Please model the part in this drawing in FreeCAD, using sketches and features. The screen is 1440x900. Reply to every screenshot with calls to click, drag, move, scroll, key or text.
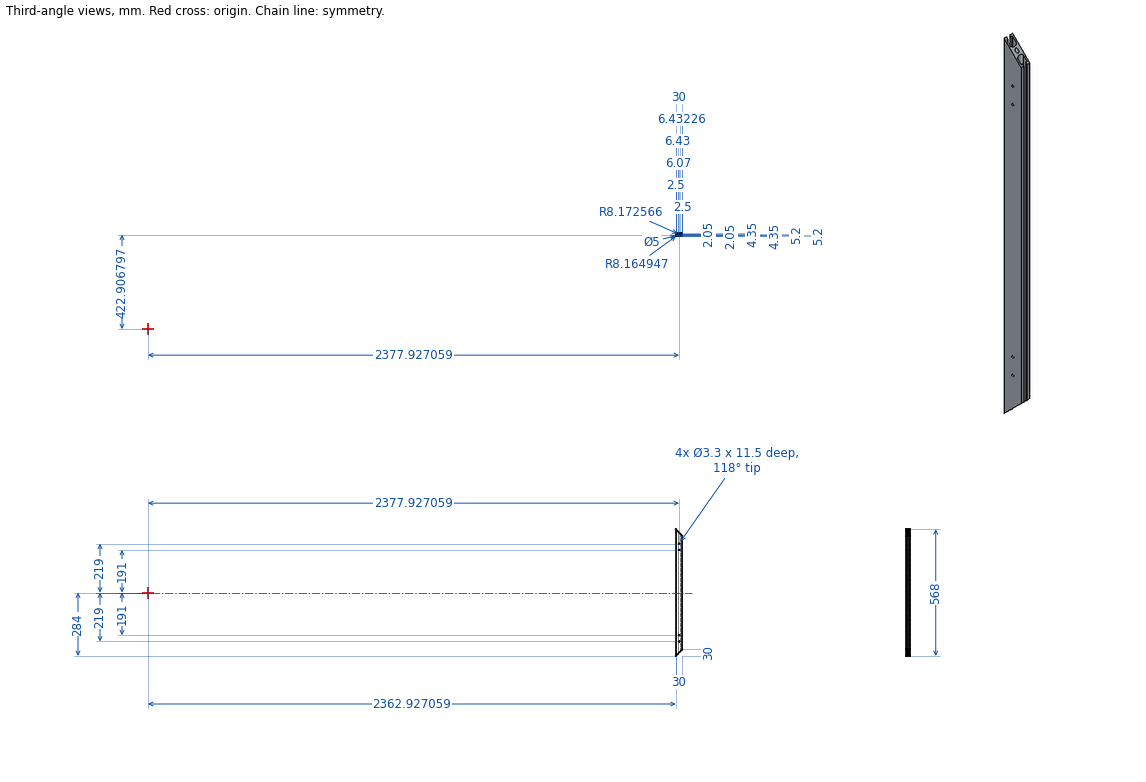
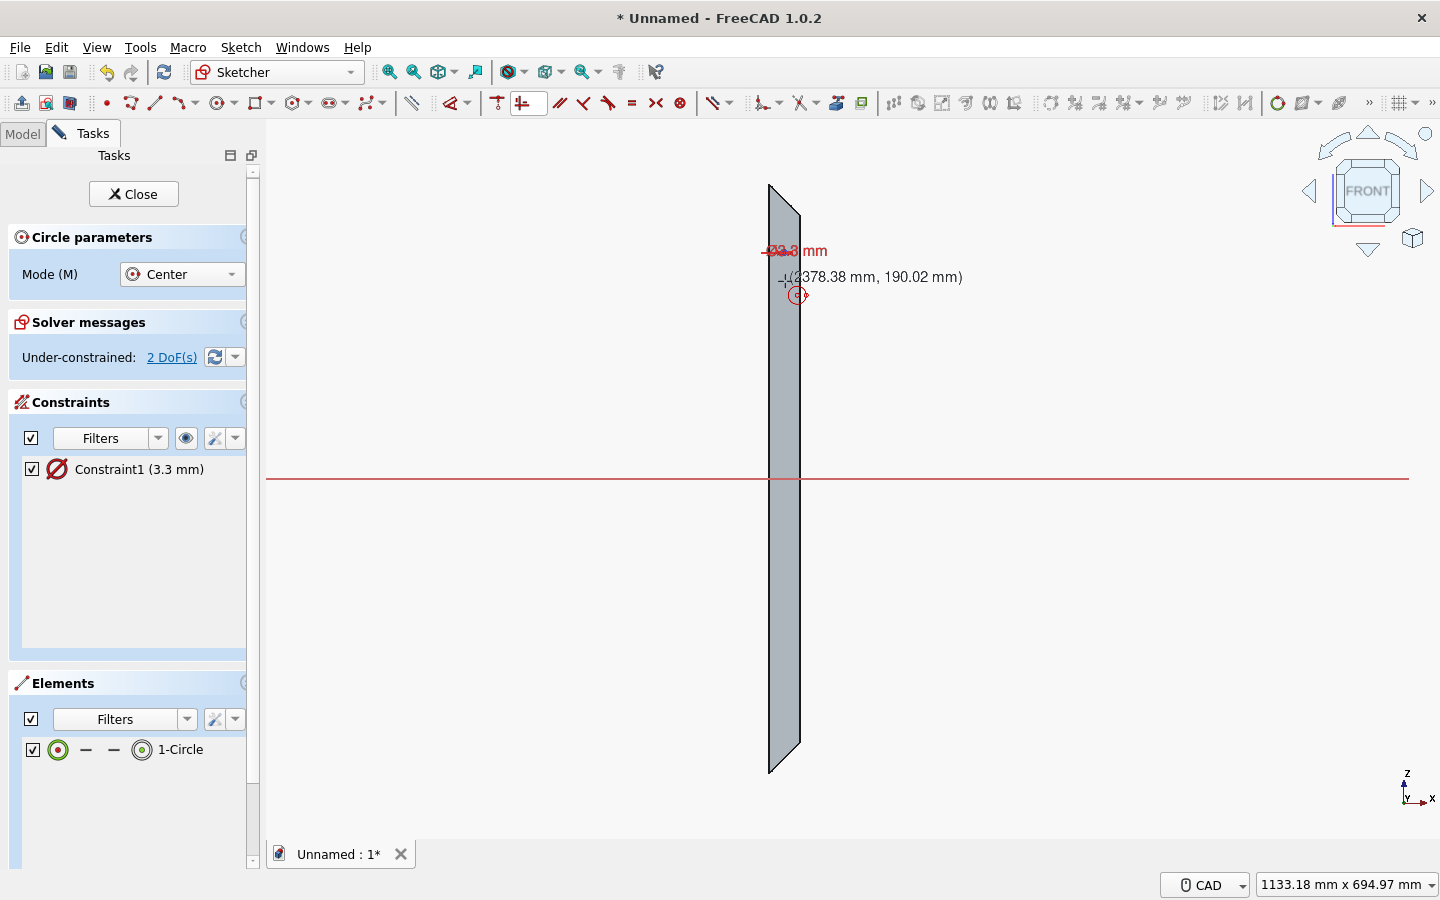
click(785, 281)
move(786, 280)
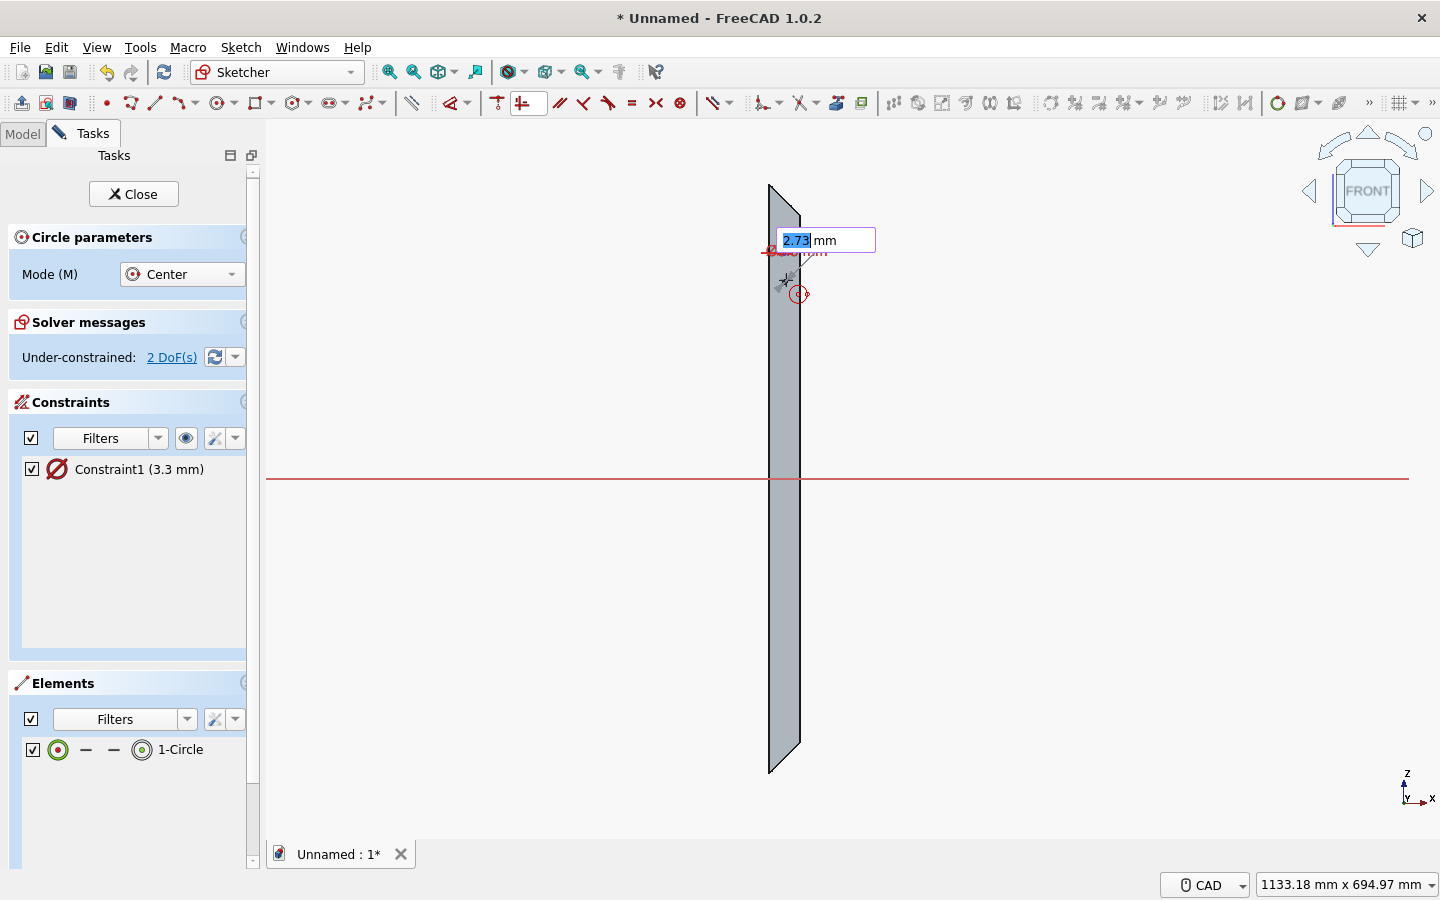
text(3.3)
key(Return)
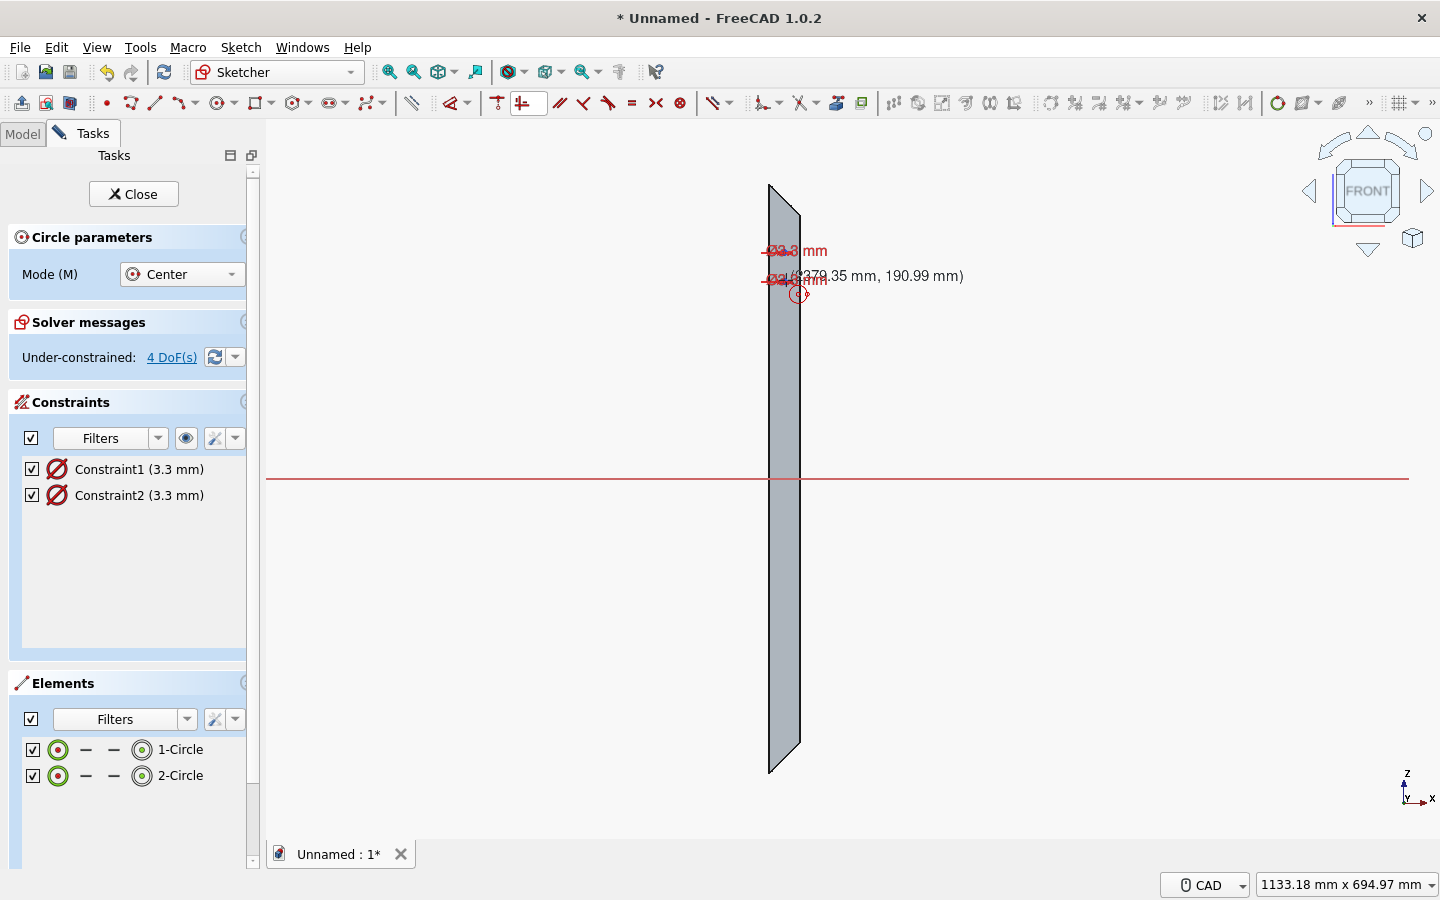
scroll(785, 677, up, 13)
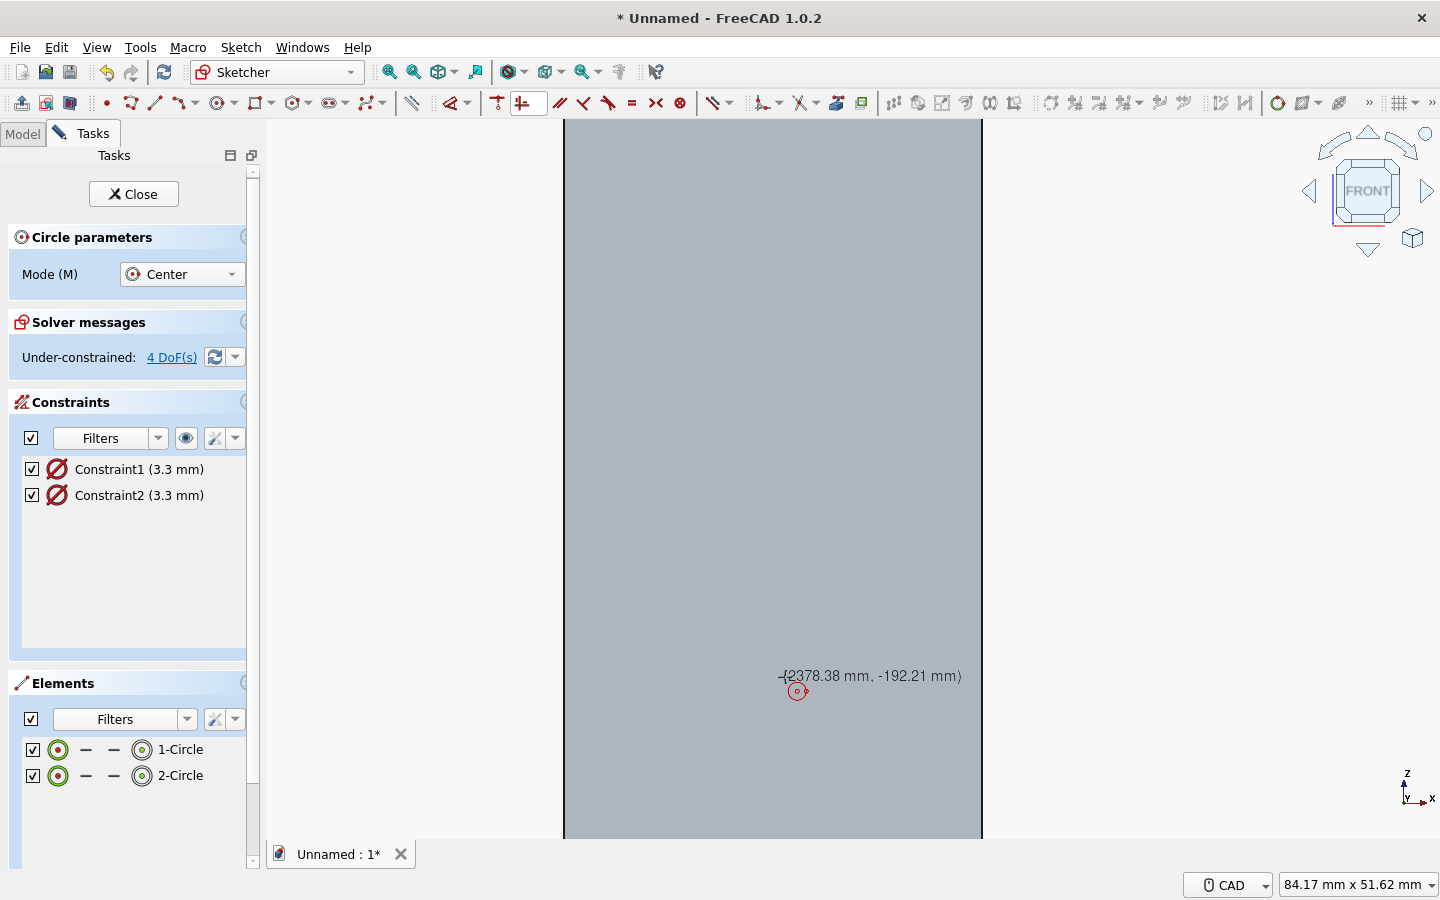
scroll(785, 678, down, 13)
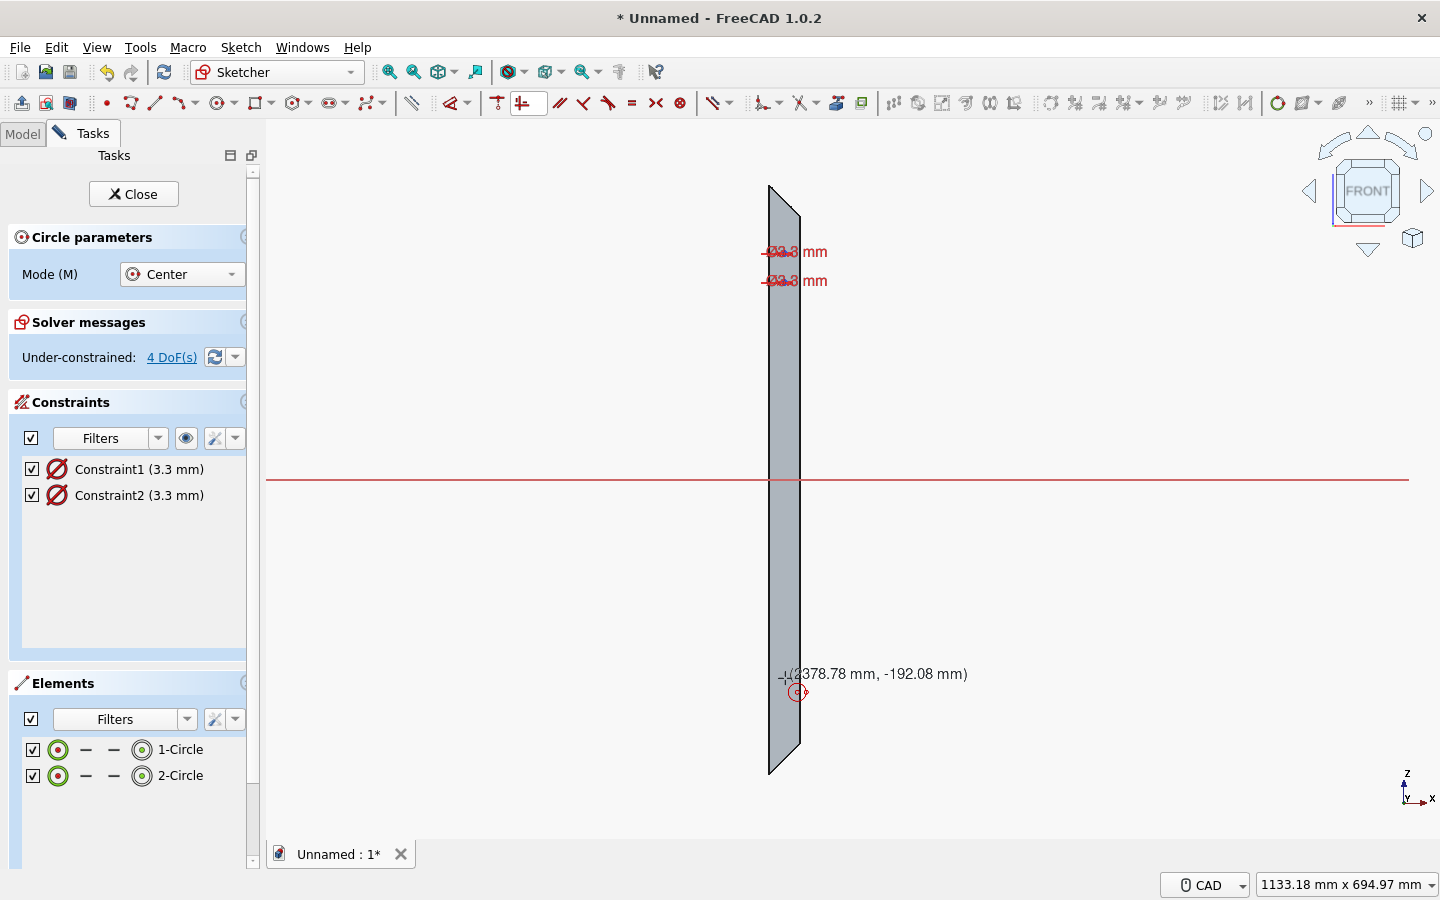
click(785, 678)
move(786, 676)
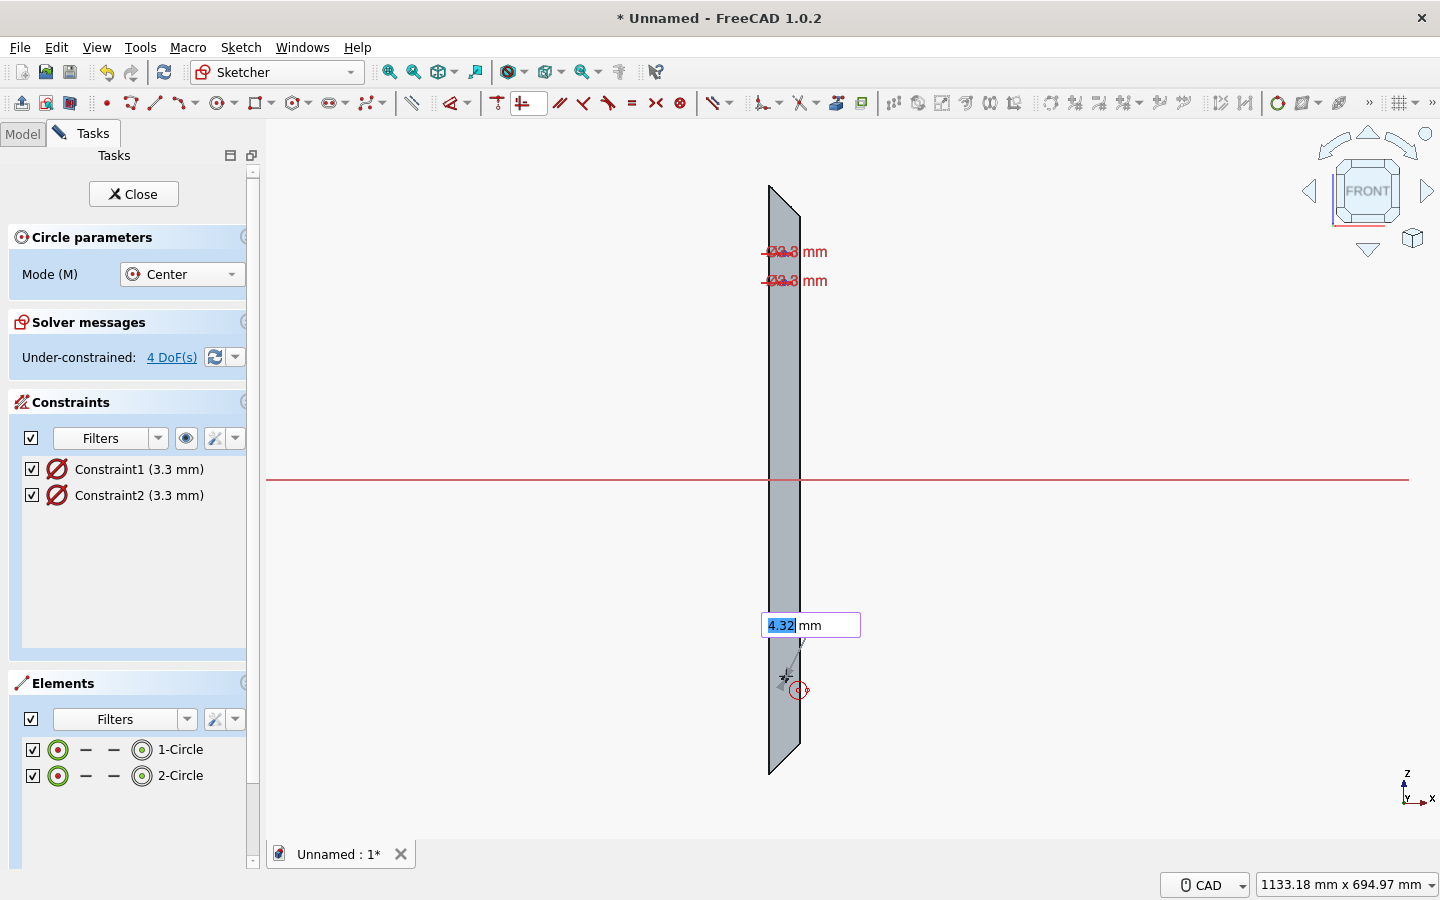
text(3.3)
key(Return)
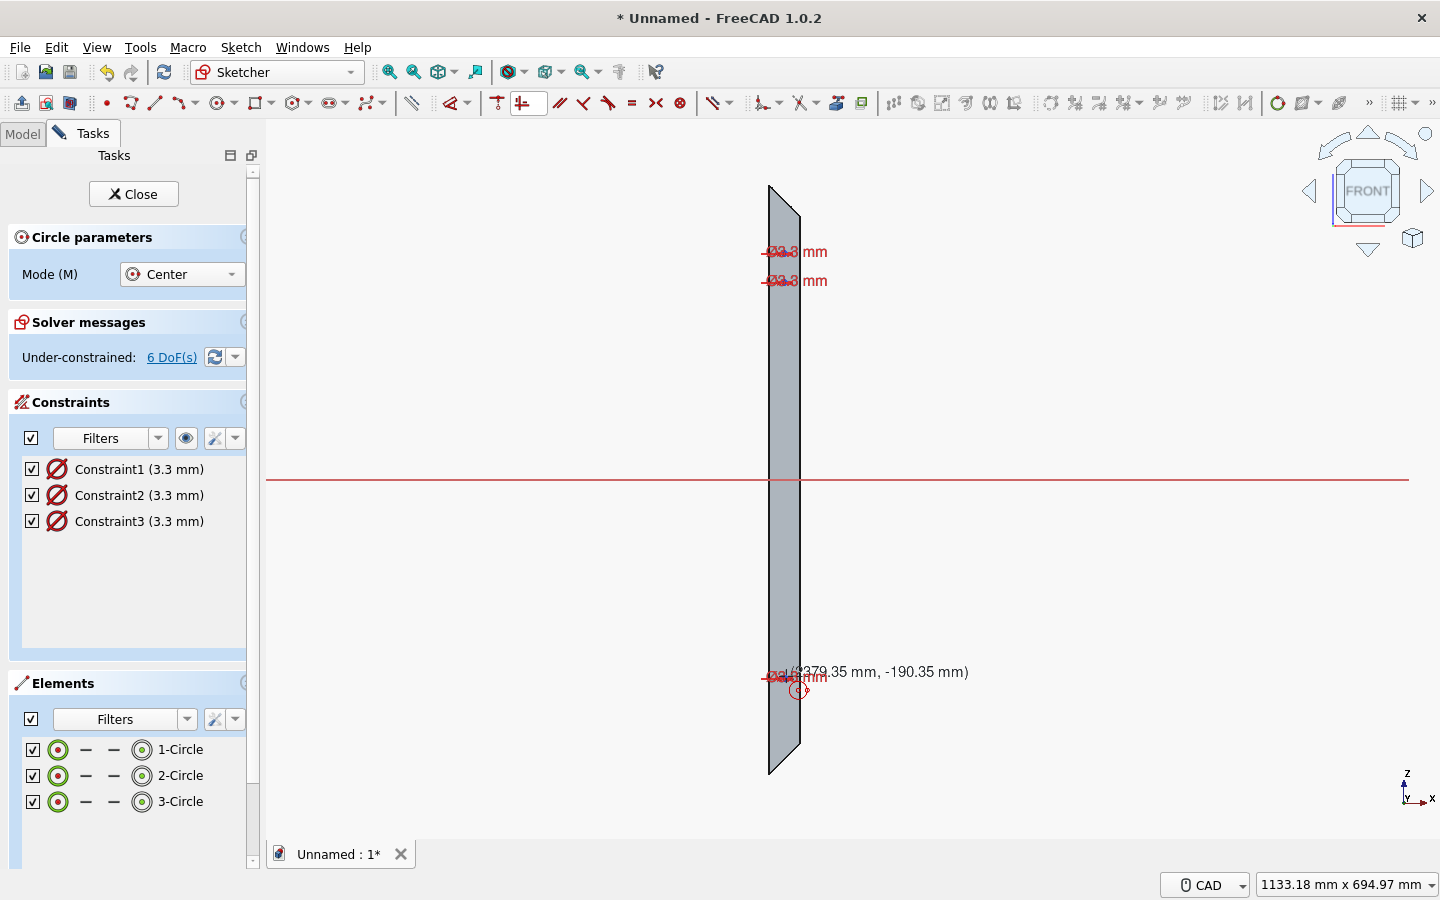
scroll(785, 707, up, 13)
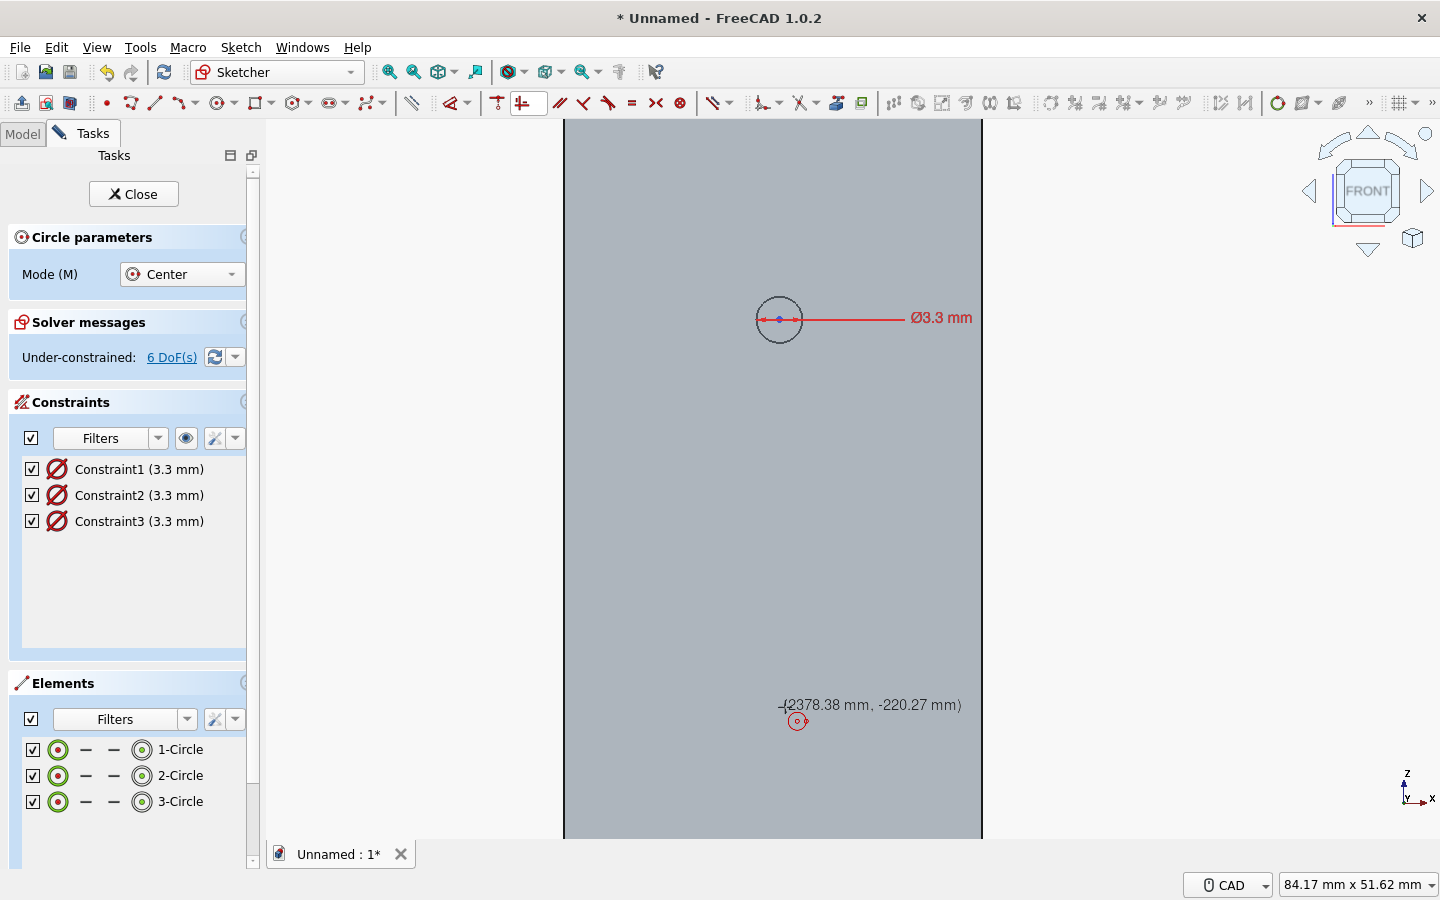
scroll(785, 707, down, 13)